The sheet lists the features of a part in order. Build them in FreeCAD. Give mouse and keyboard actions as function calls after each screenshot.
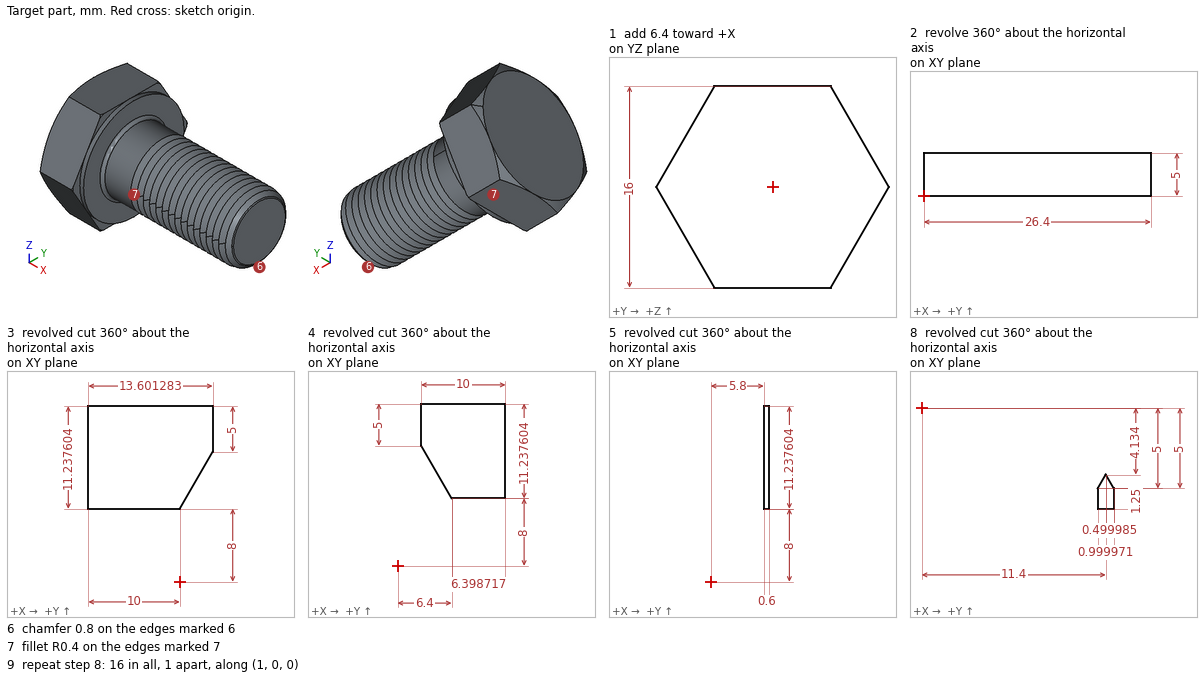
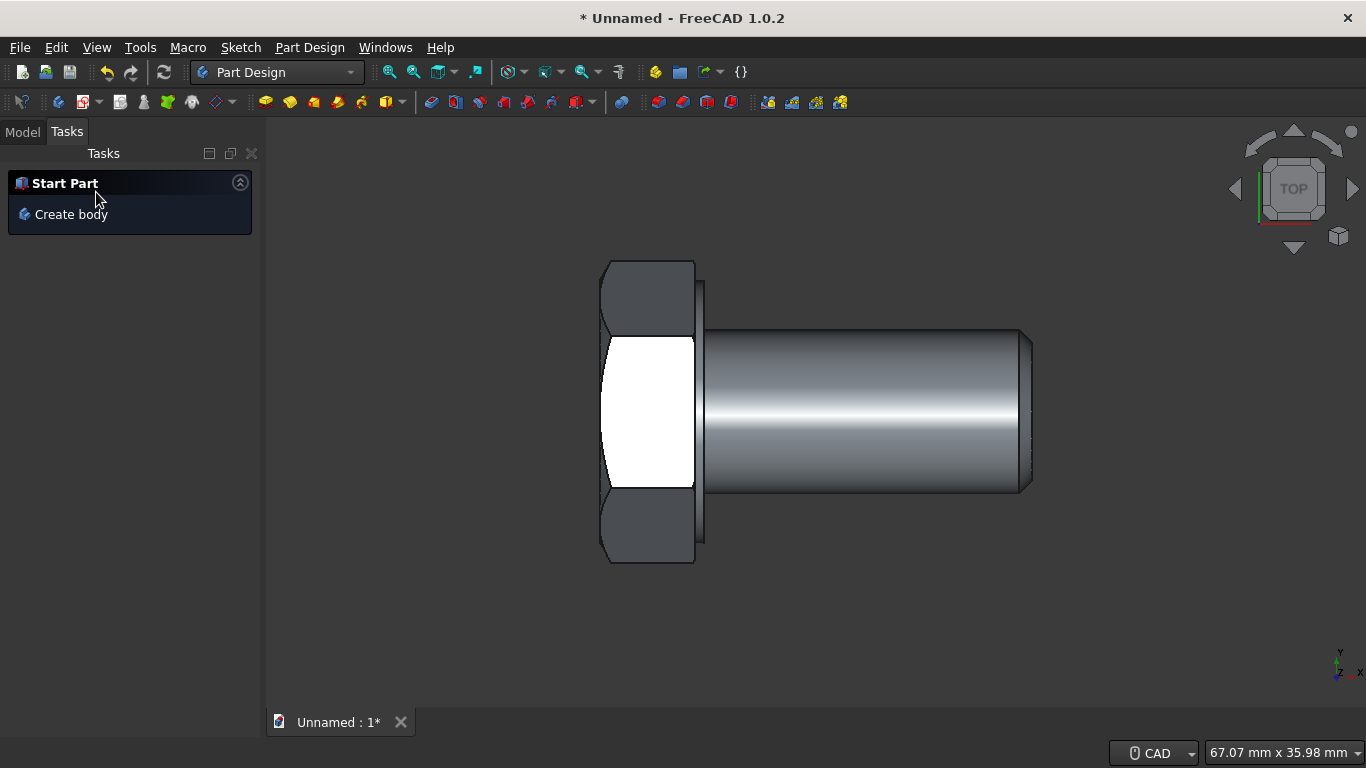
key(1)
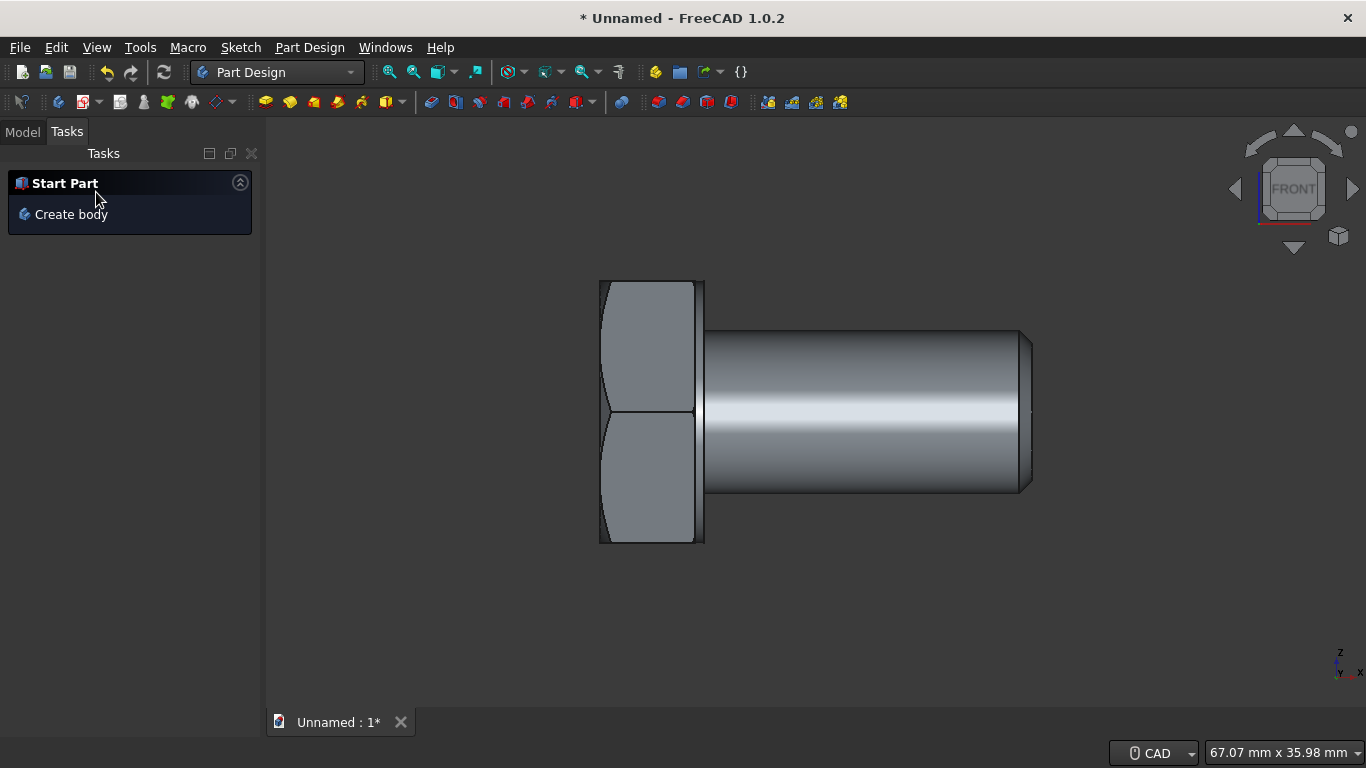
click(390, 72)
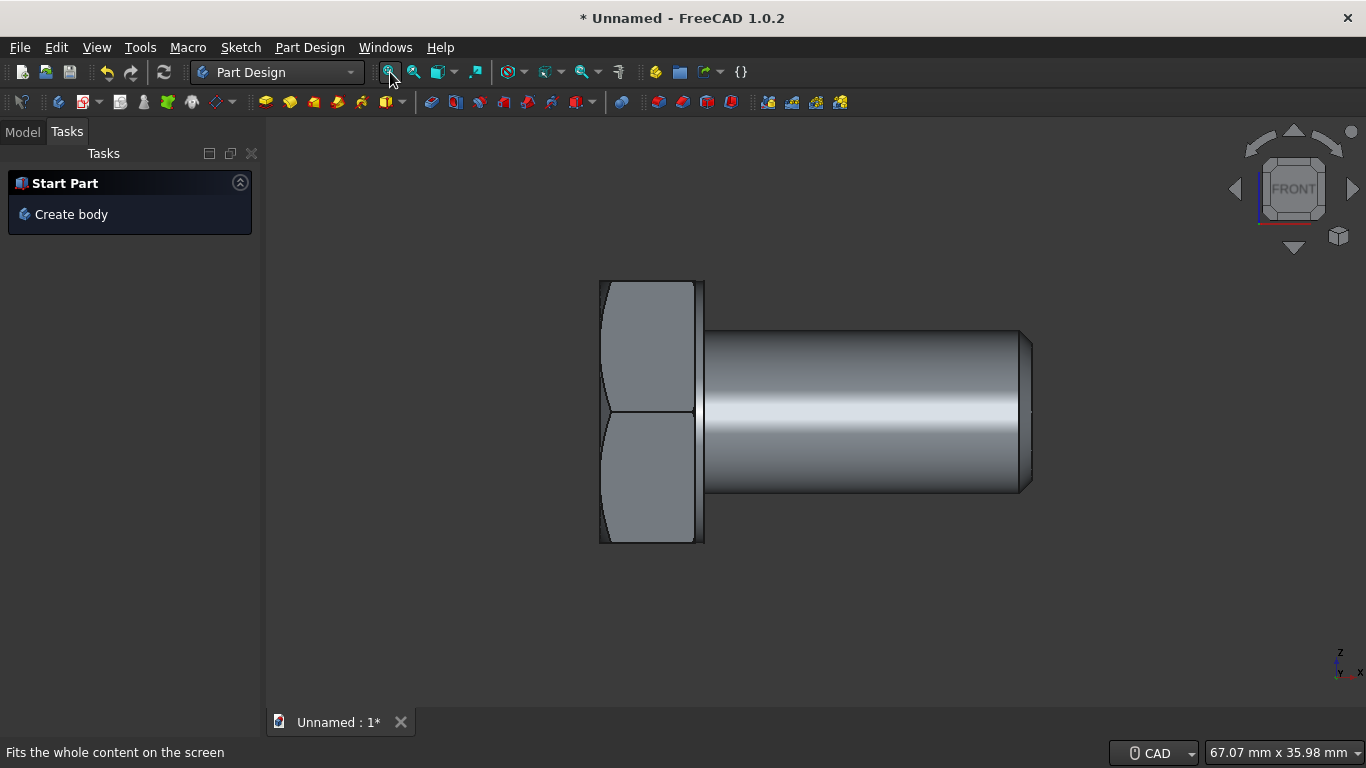
key(3)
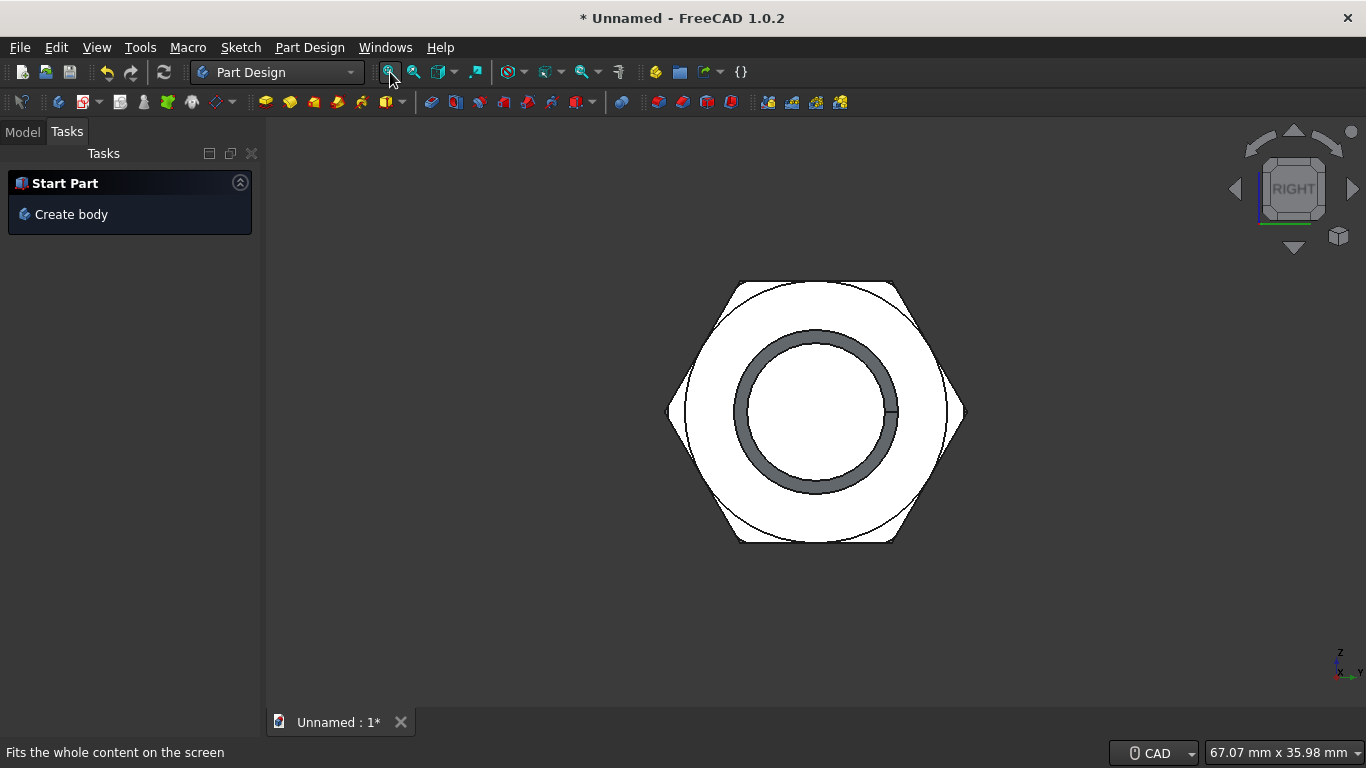
click(390, 72)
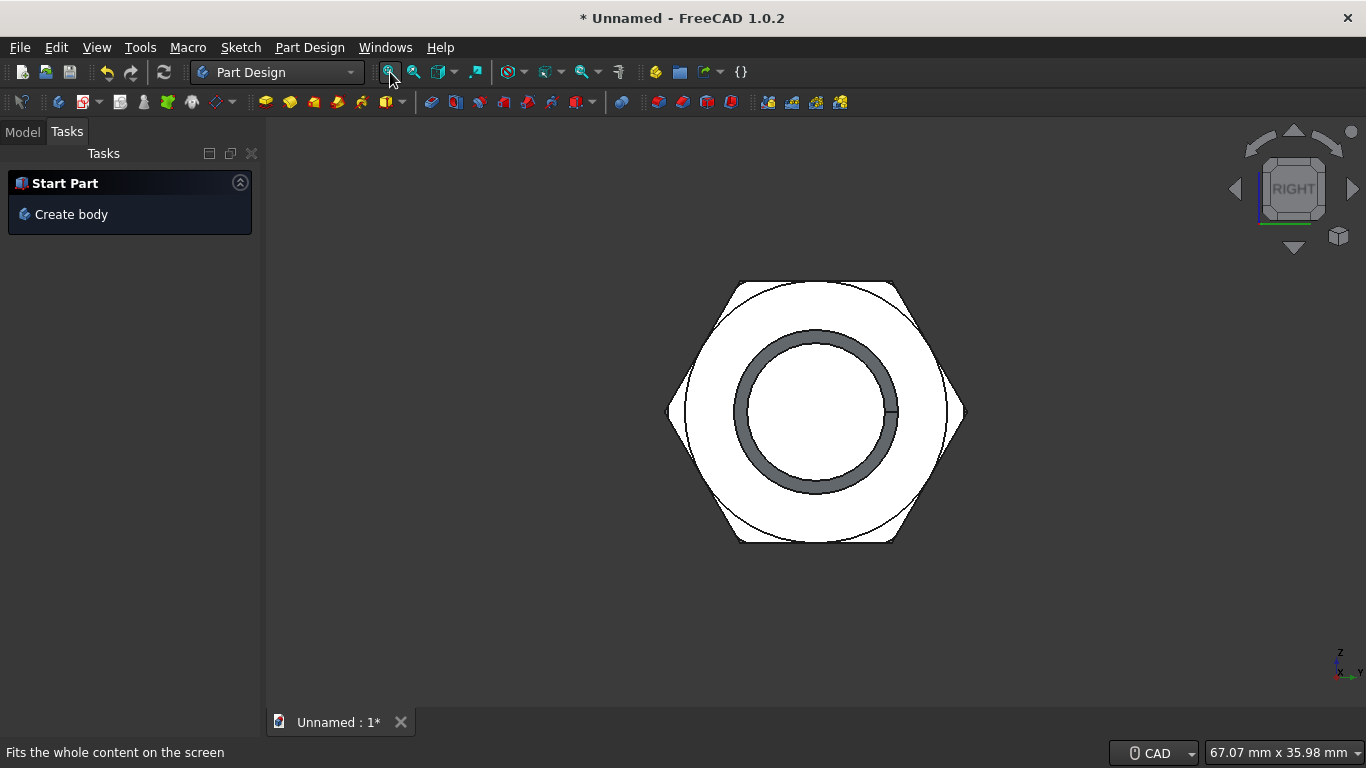
key(5)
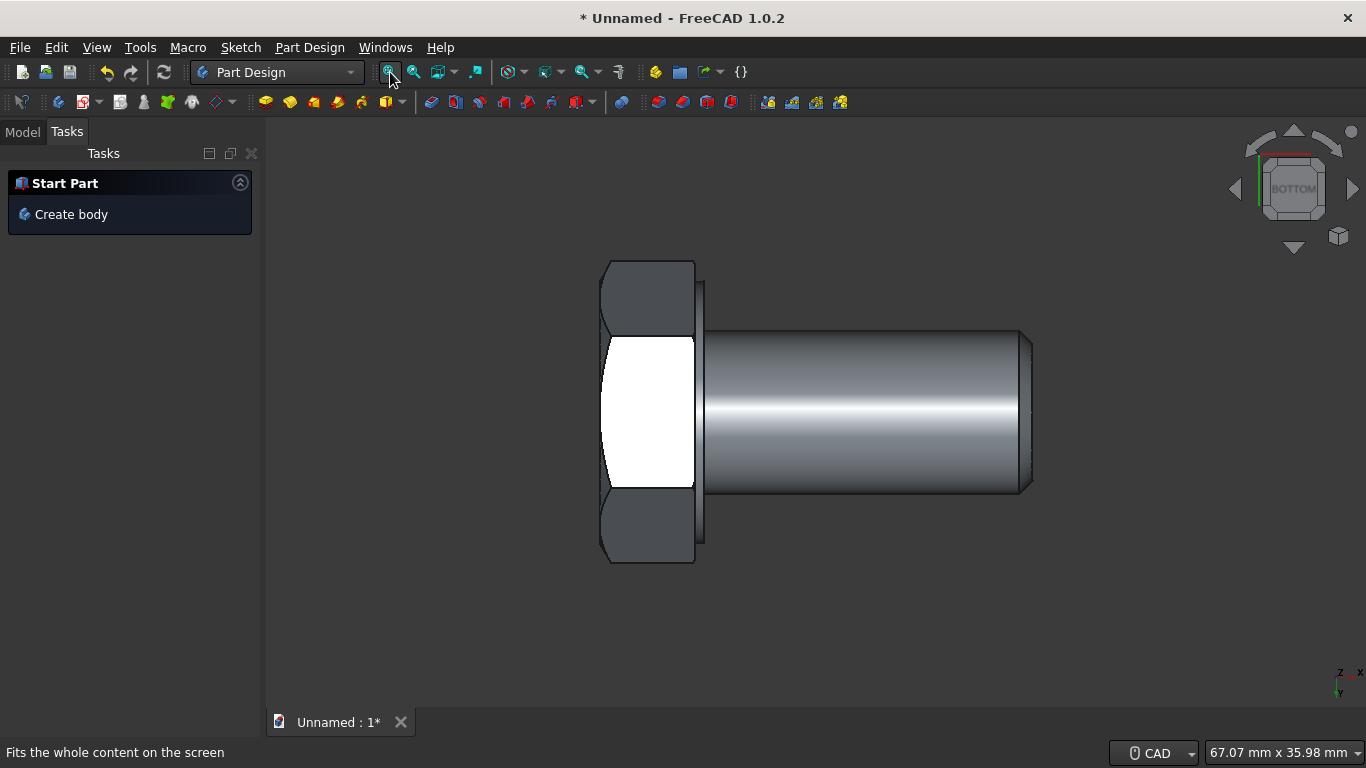
key(4)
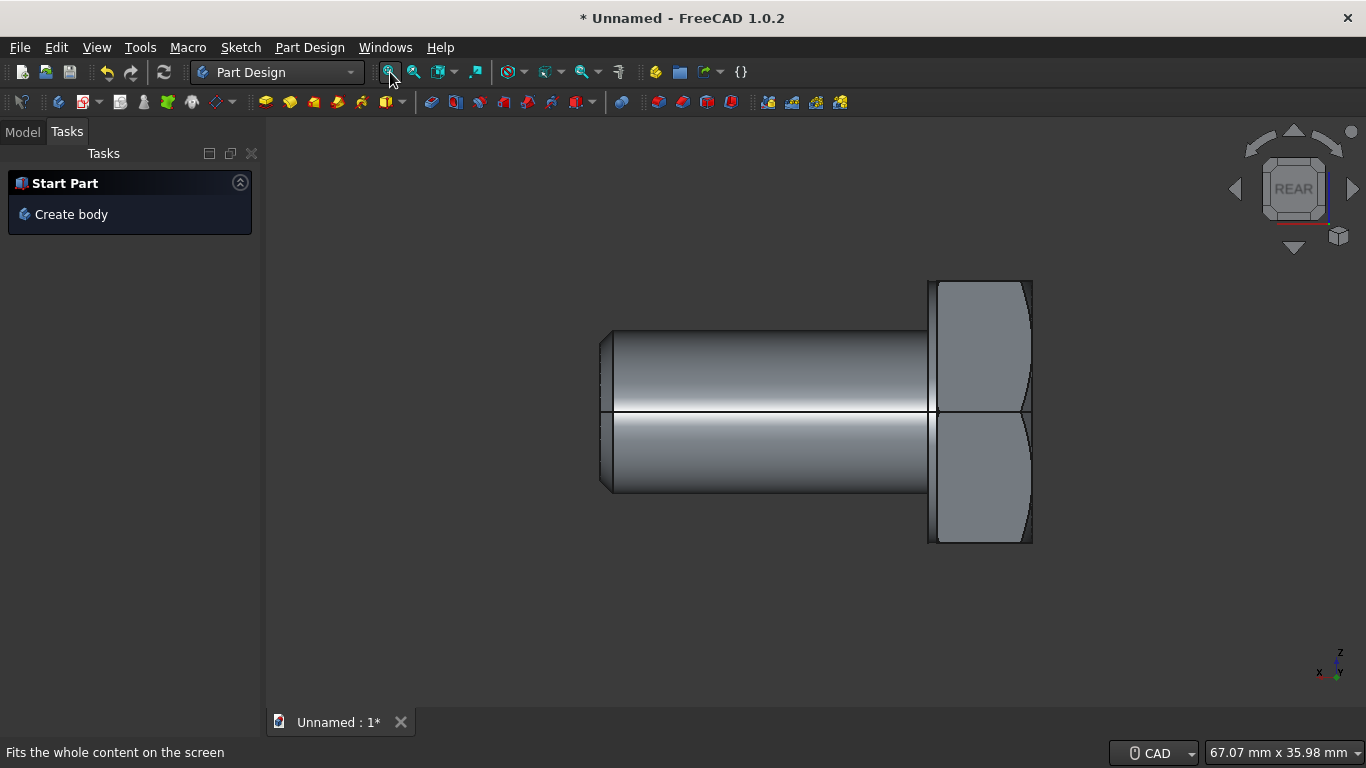
key(v)
key(f)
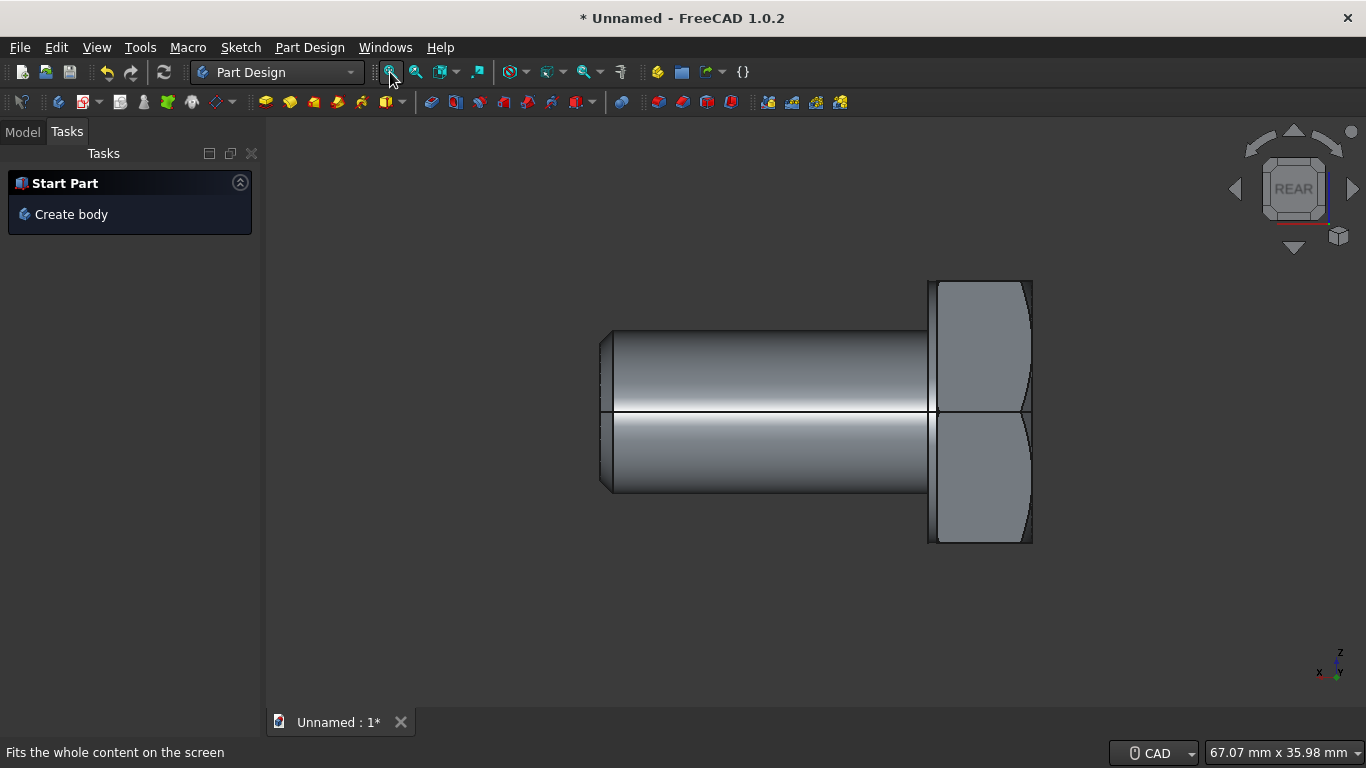
key(6)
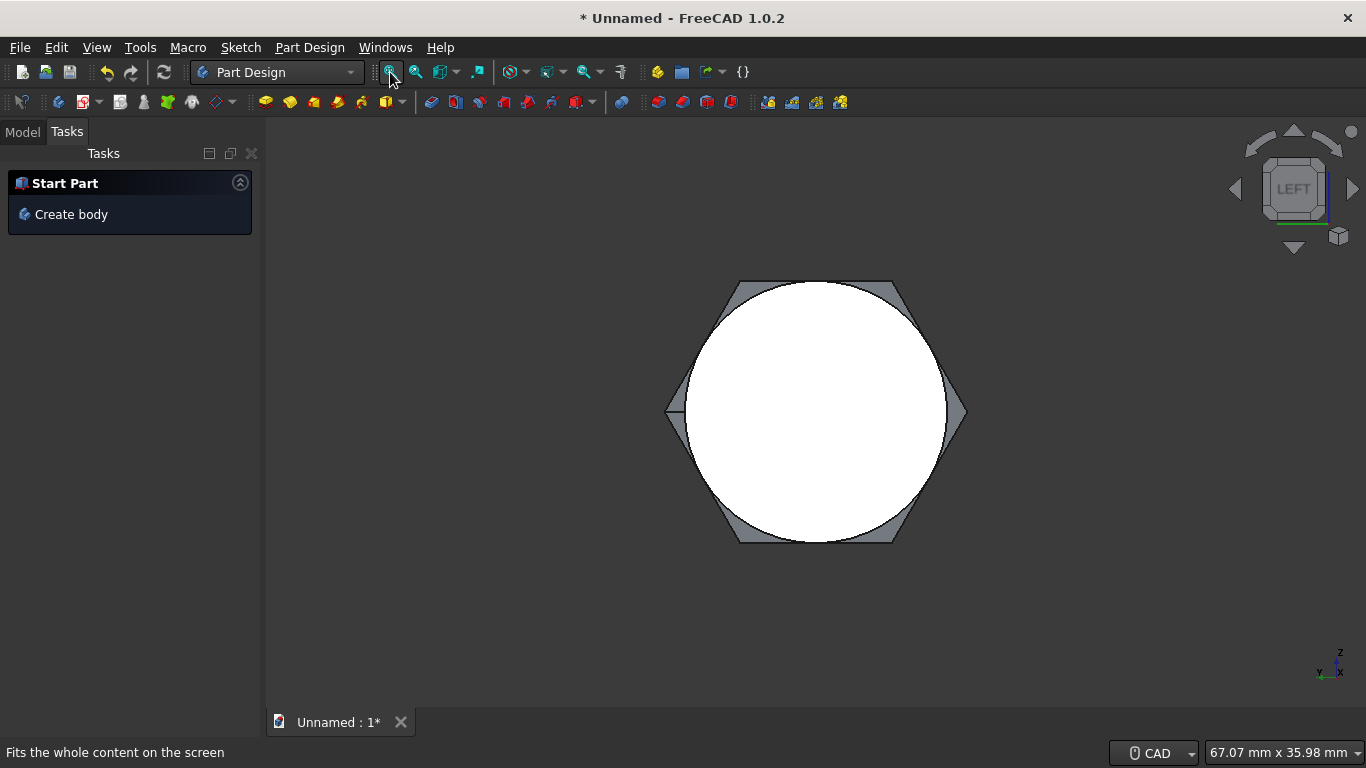
key(v)
key(f)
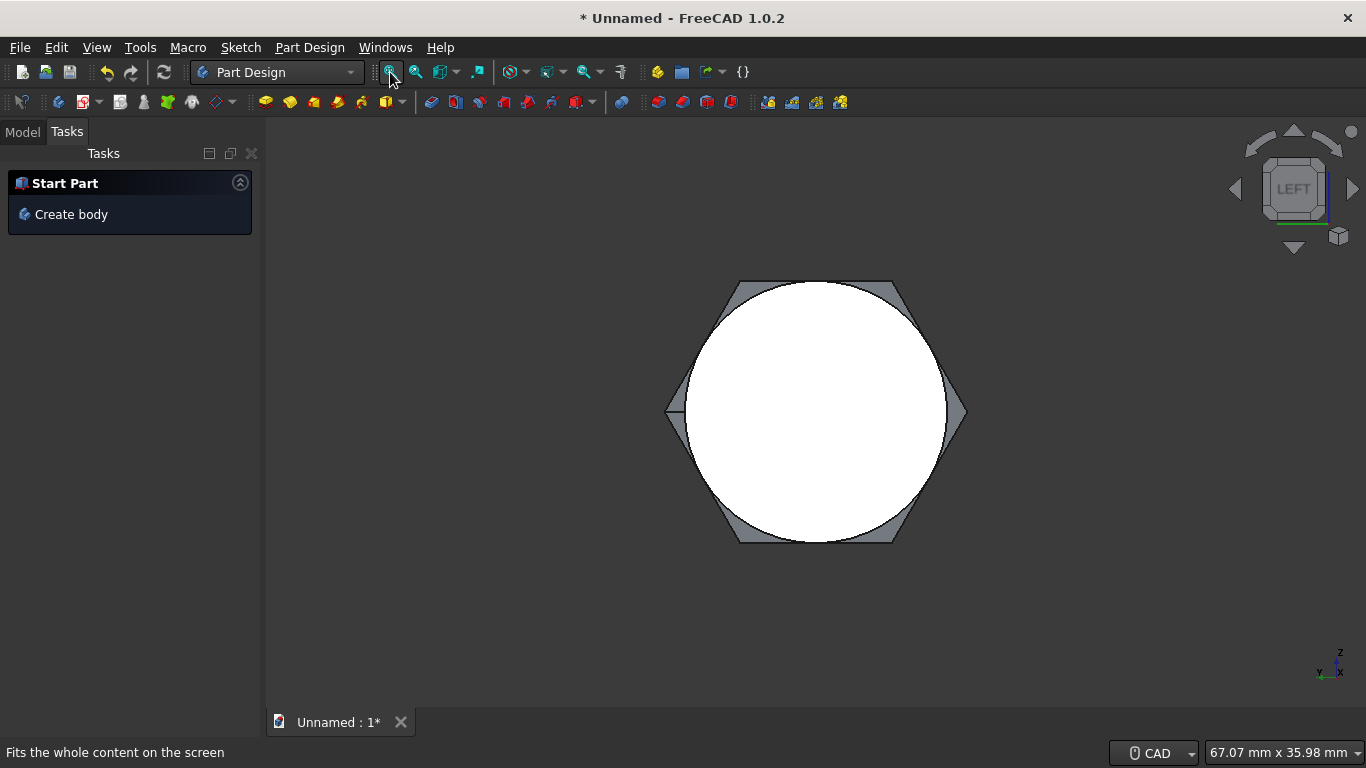
key(v)
key(3)